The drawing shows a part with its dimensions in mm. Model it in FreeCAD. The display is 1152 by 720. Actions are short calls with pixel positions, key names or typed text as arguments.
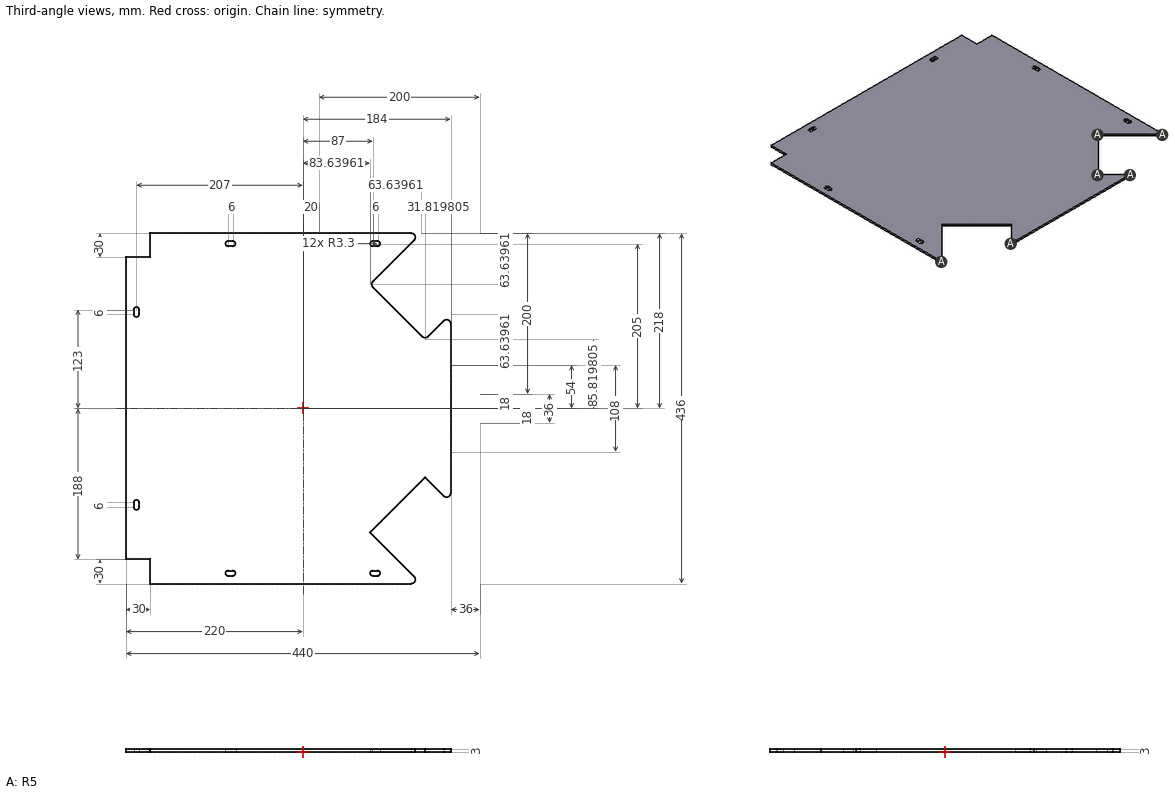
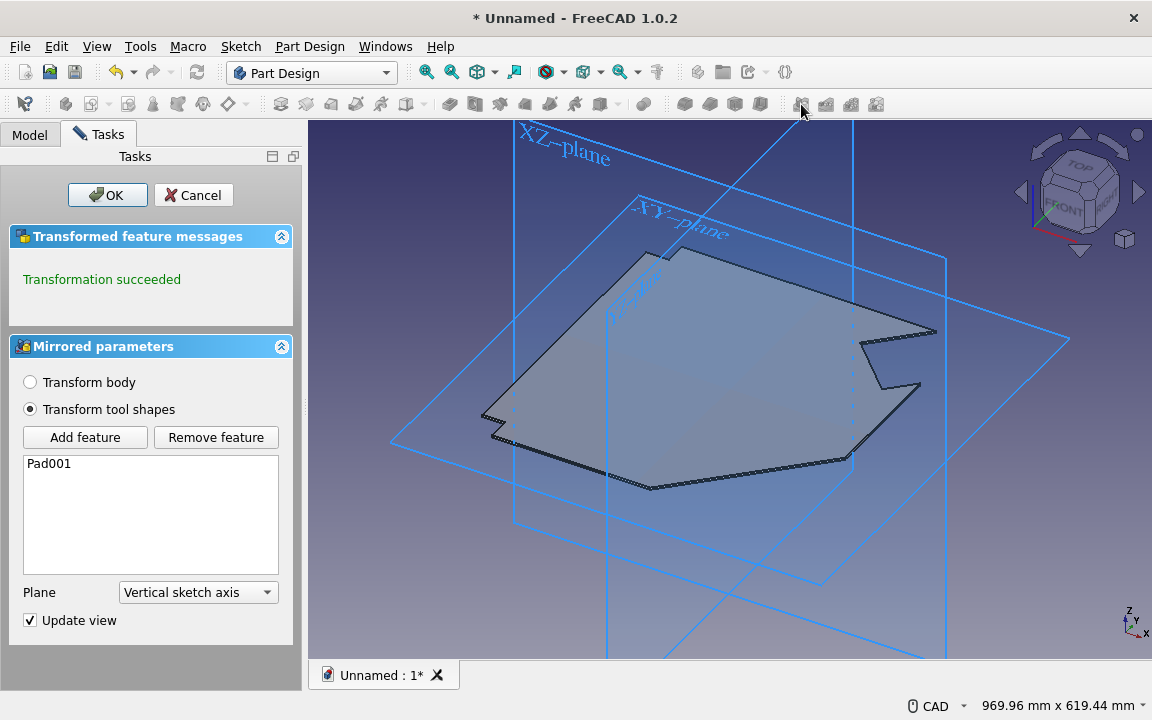
click(199, 592)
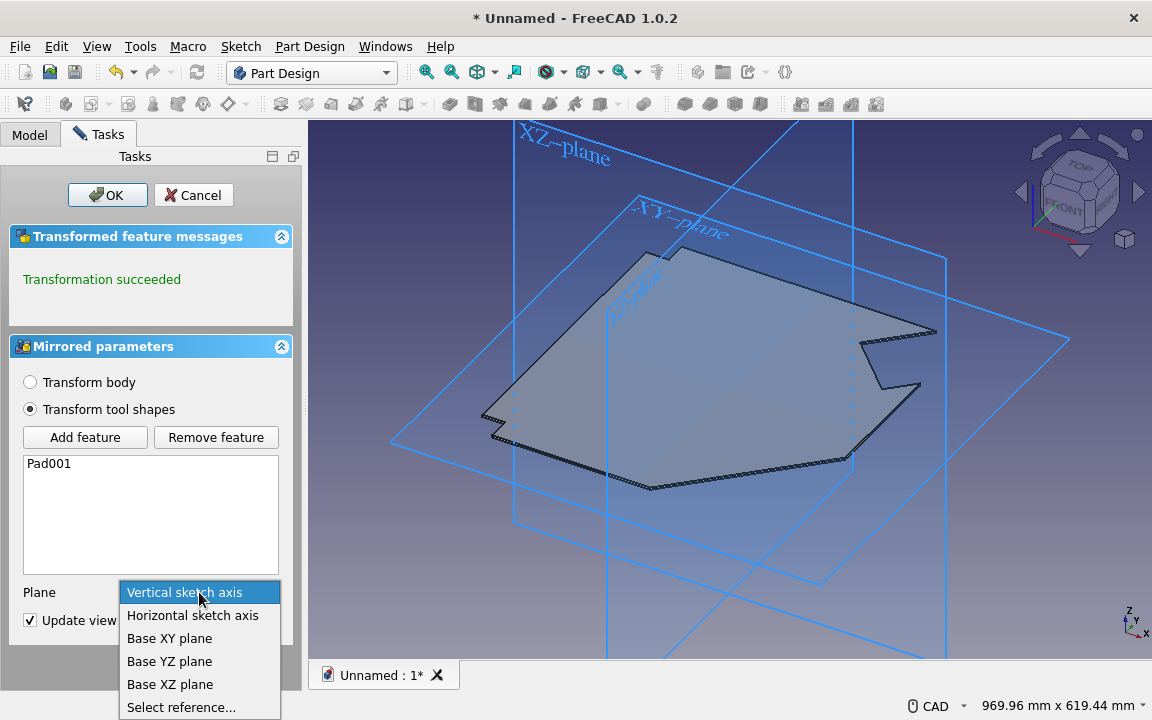
click(198, 684)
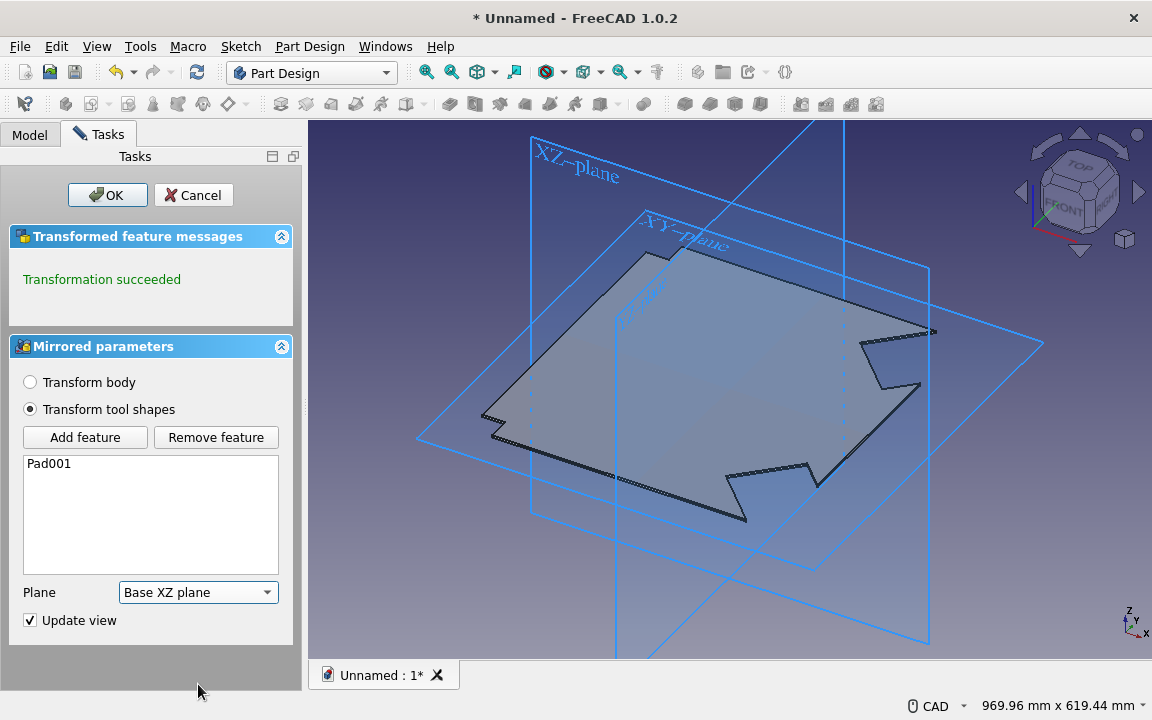
click(108, 195)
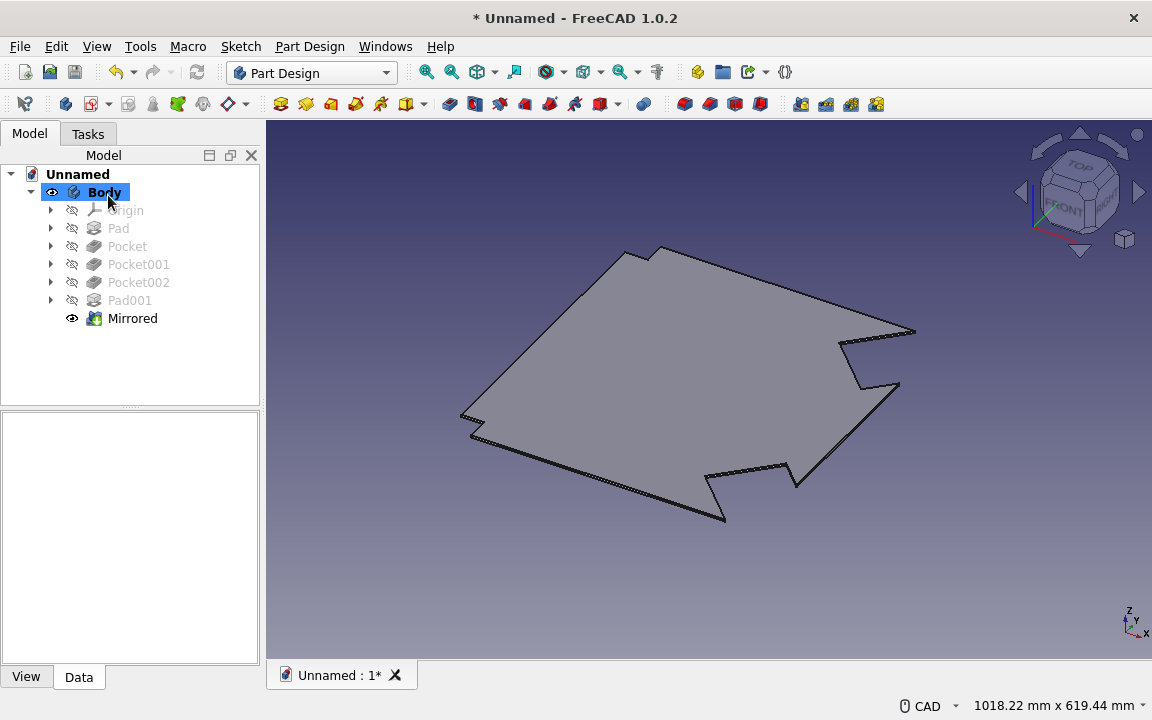
scroll(839, 343, up, 14)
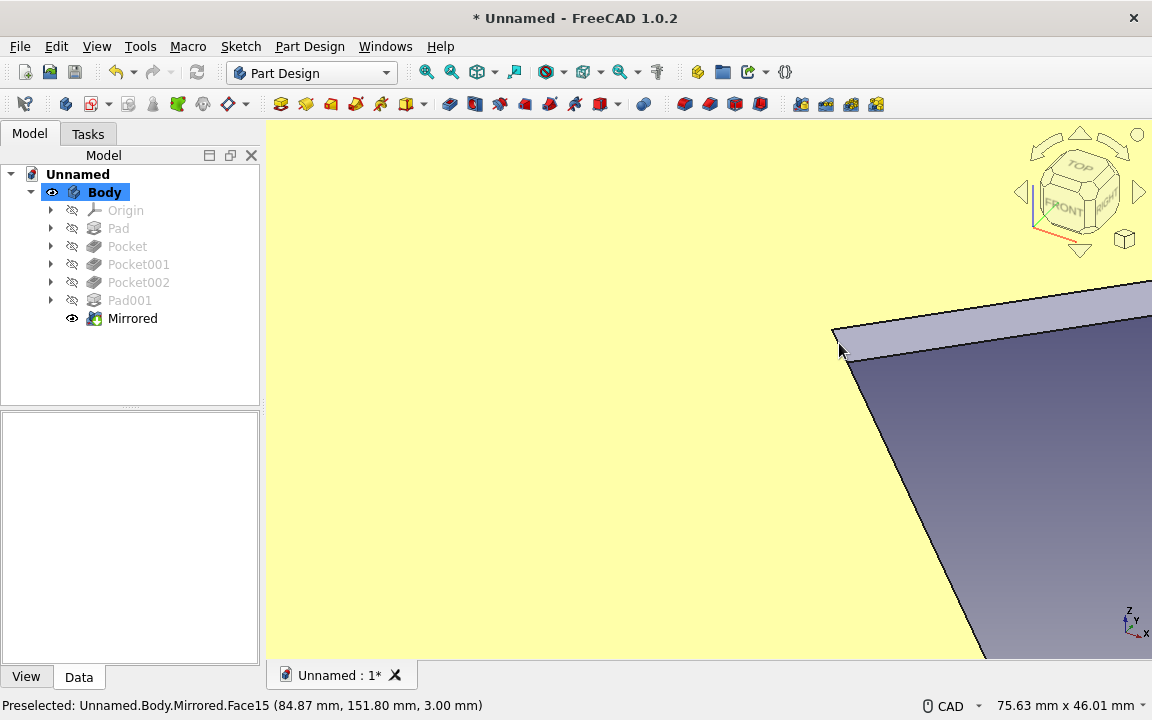
click(427, 72)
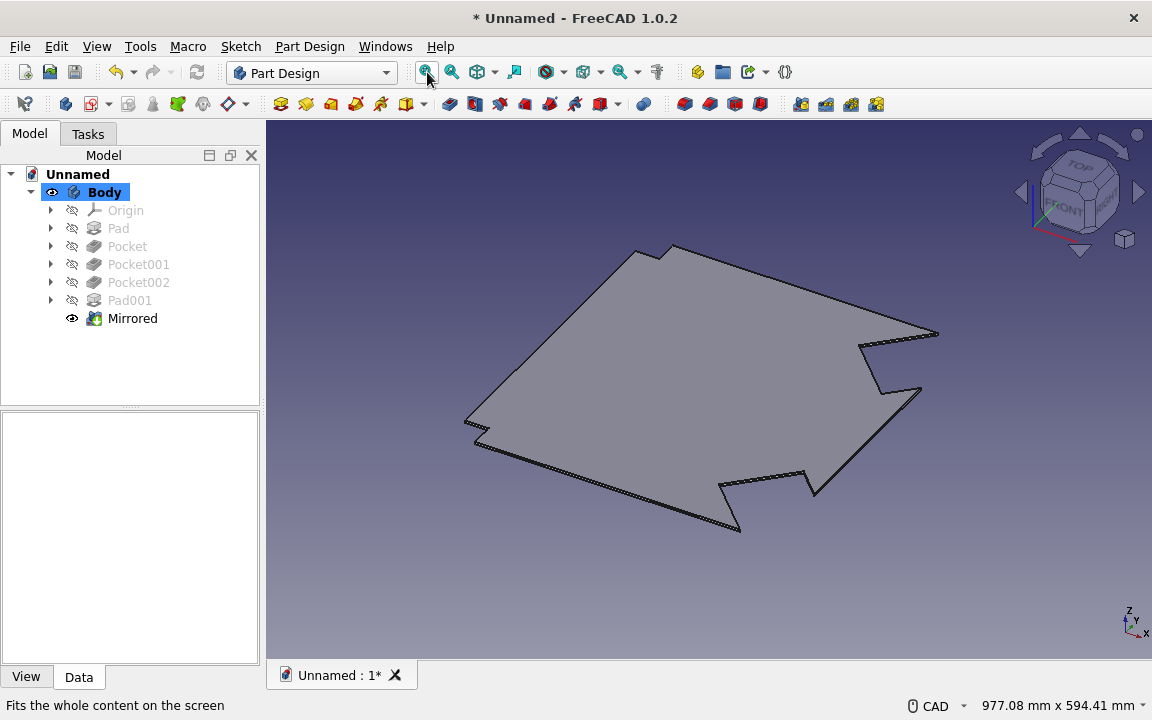
key(0)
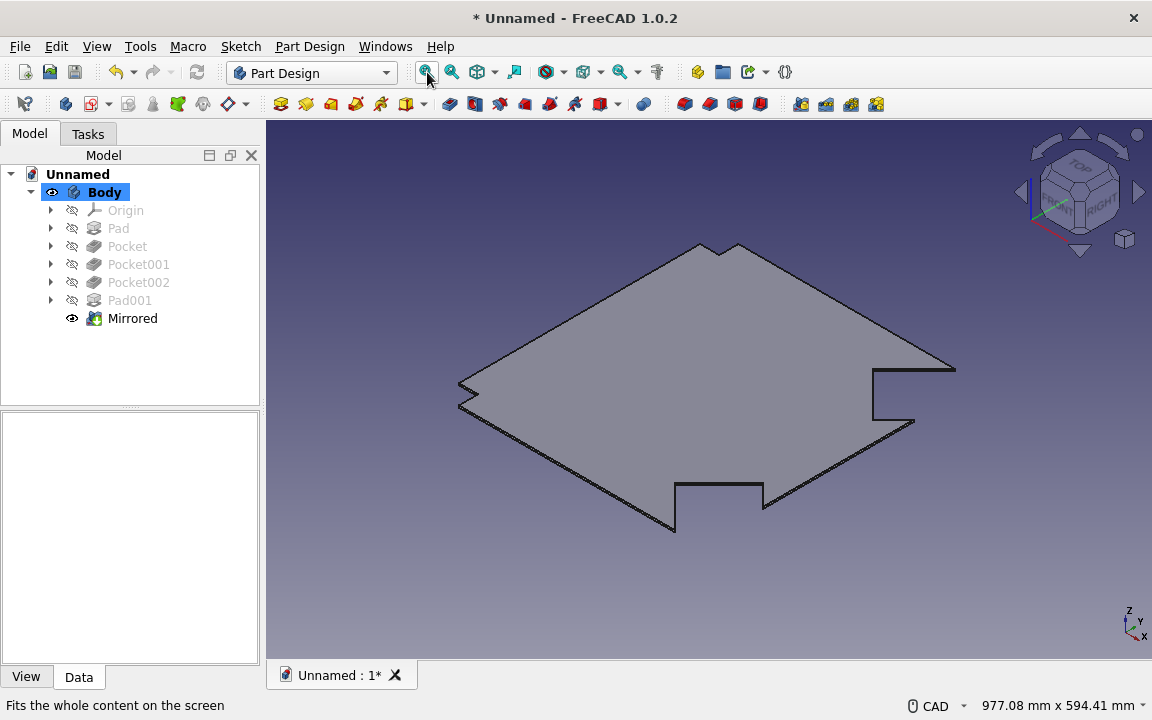
scroll(873, 369, up, 14)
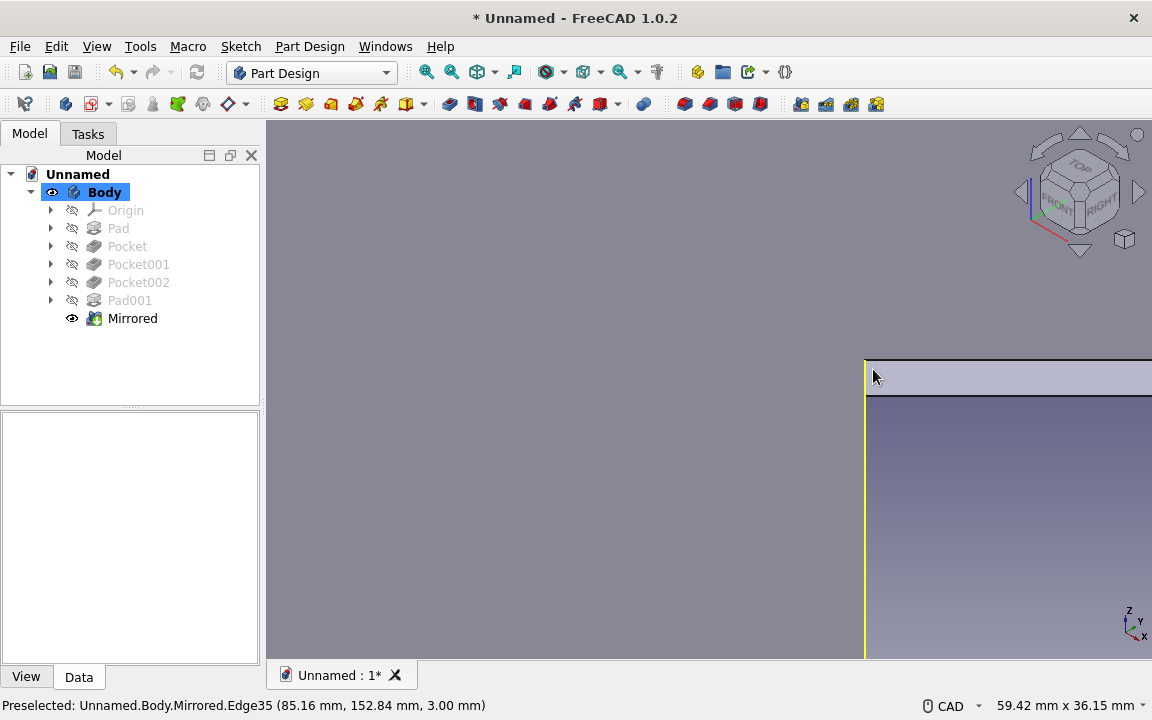
key(v)
key(f)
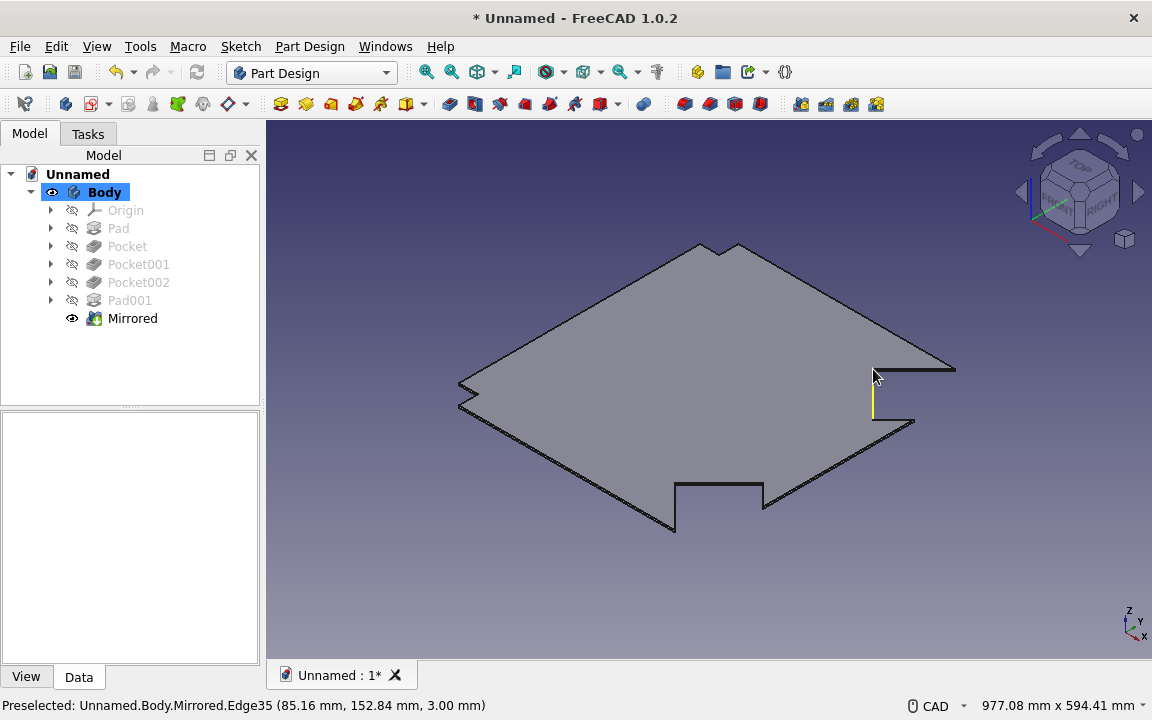
key(2)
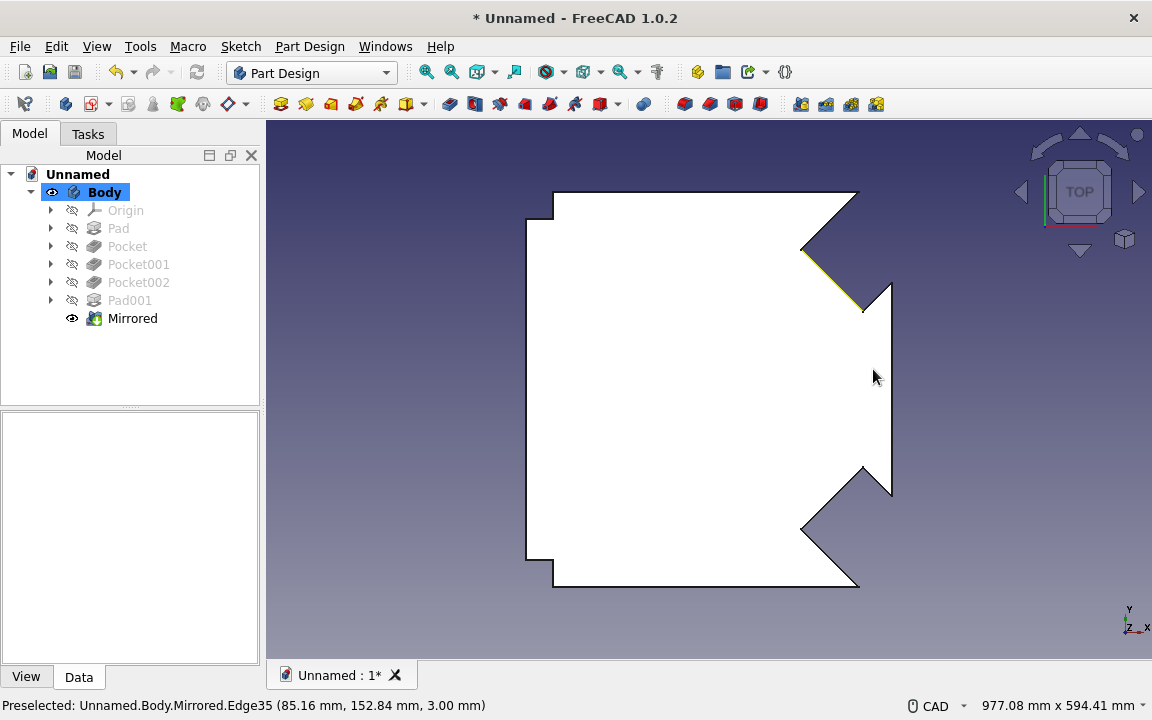
scroll(801, 249, up, 14)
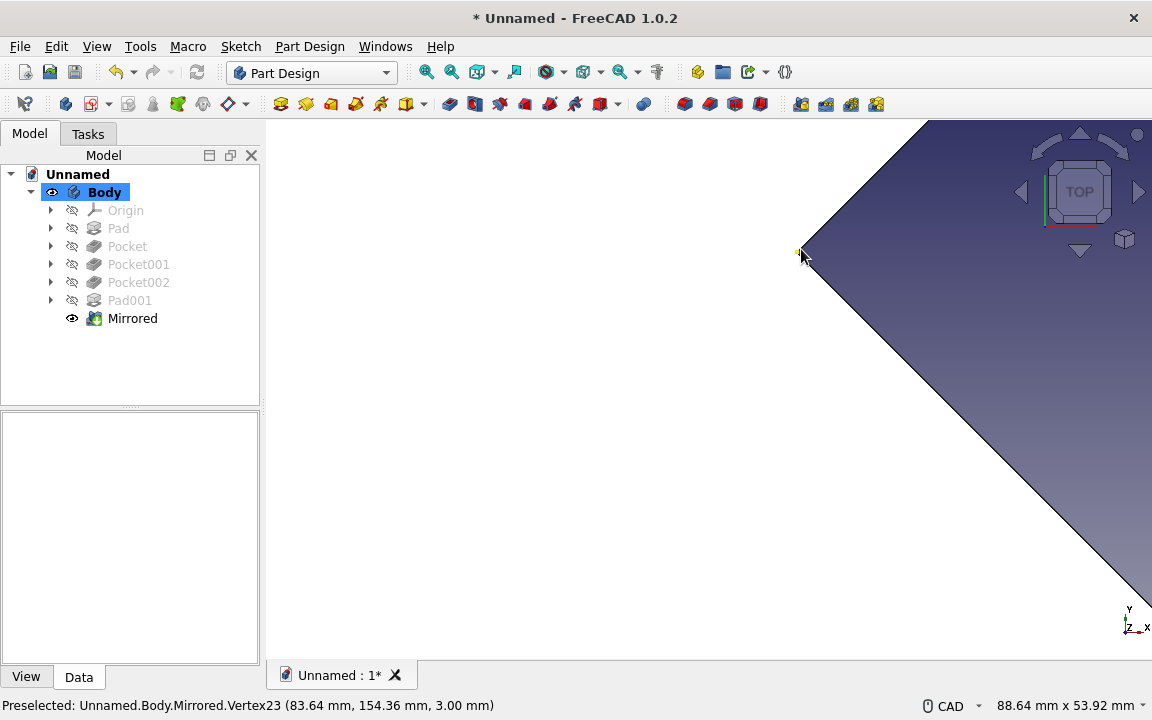
key(v)
key(f)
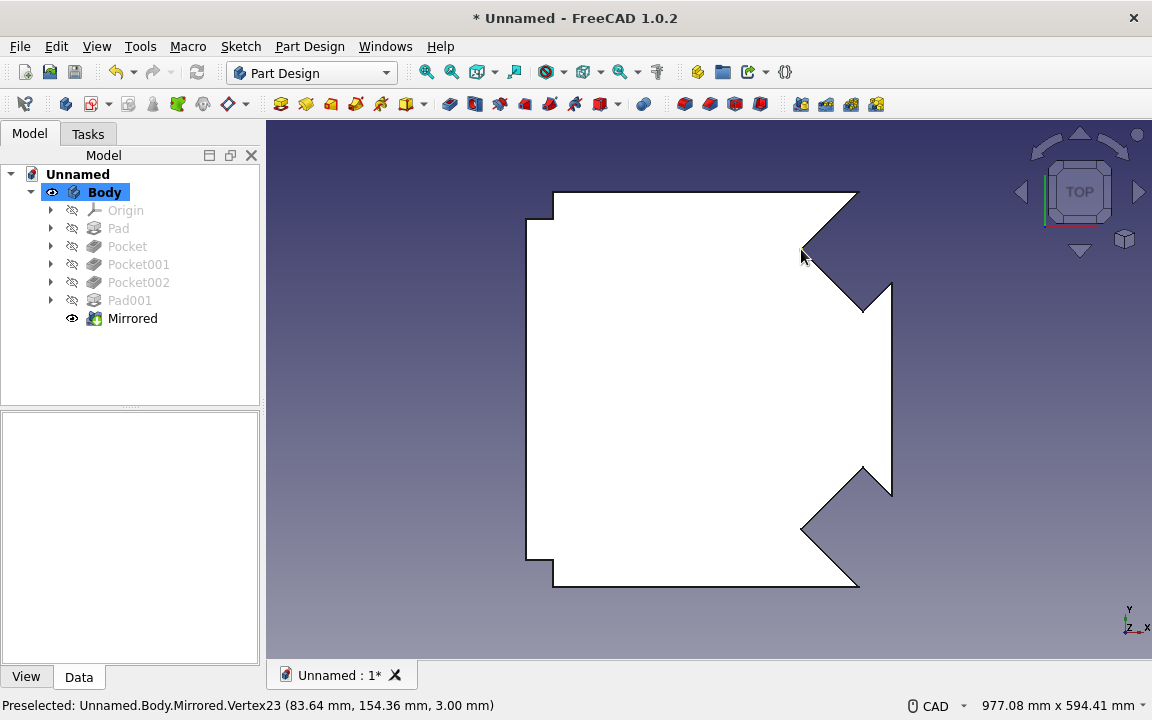
key(1)